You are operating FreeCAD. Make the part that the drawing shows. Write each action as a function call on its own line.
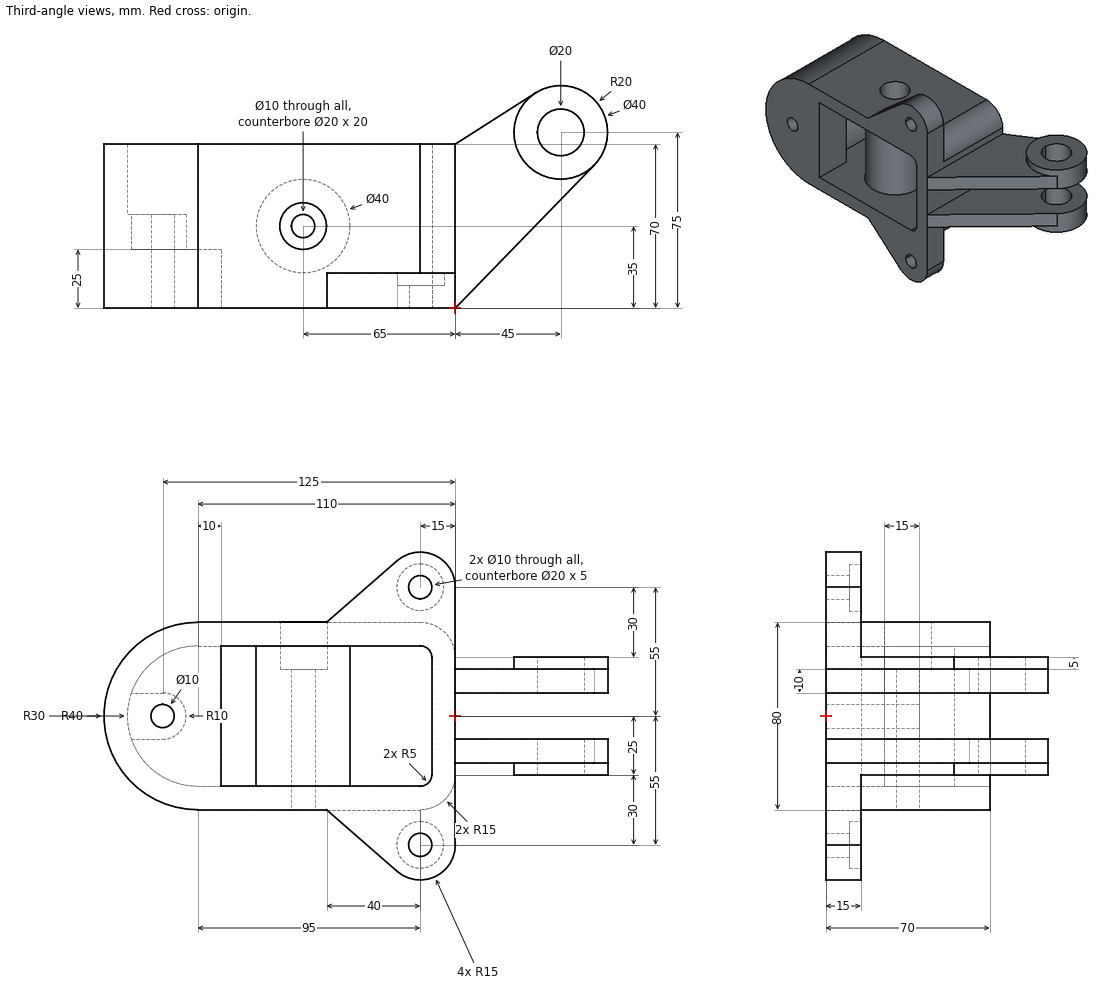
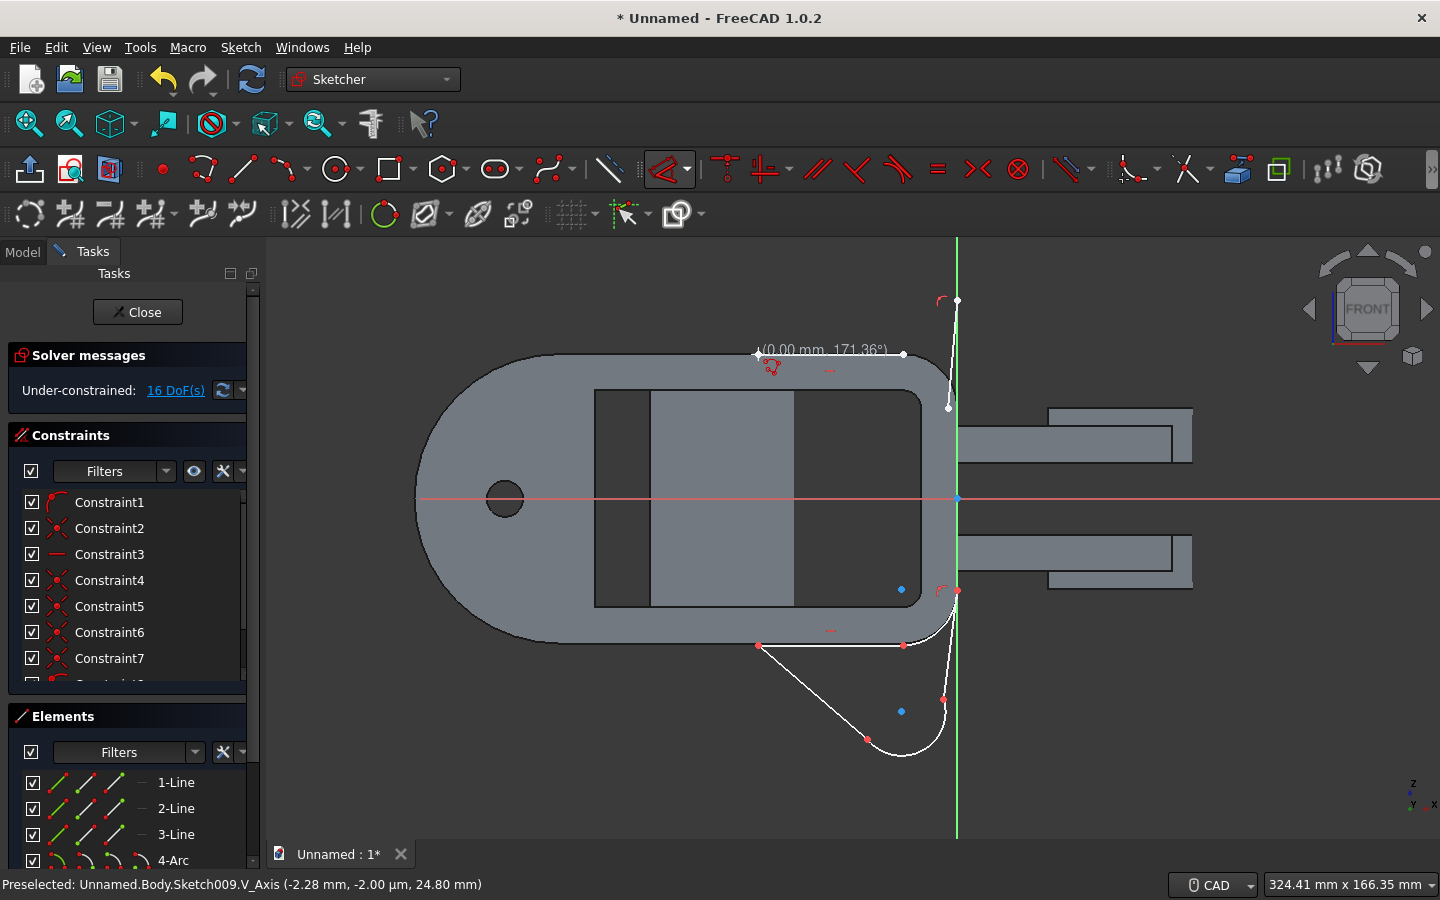
scroll(453, 715, down, 1)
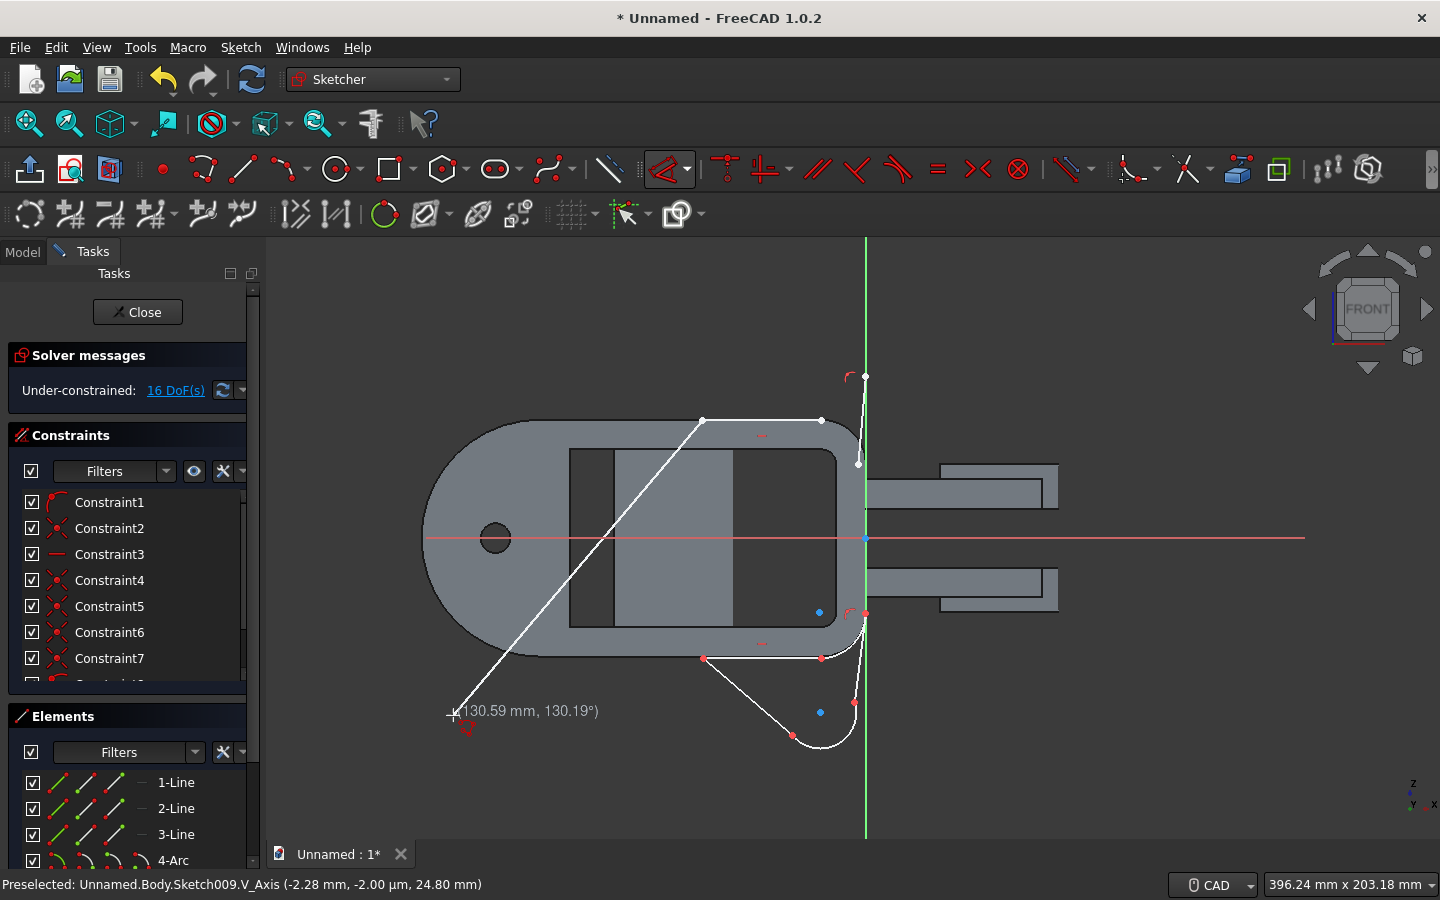
click(792, 342)
right_click(792, 342)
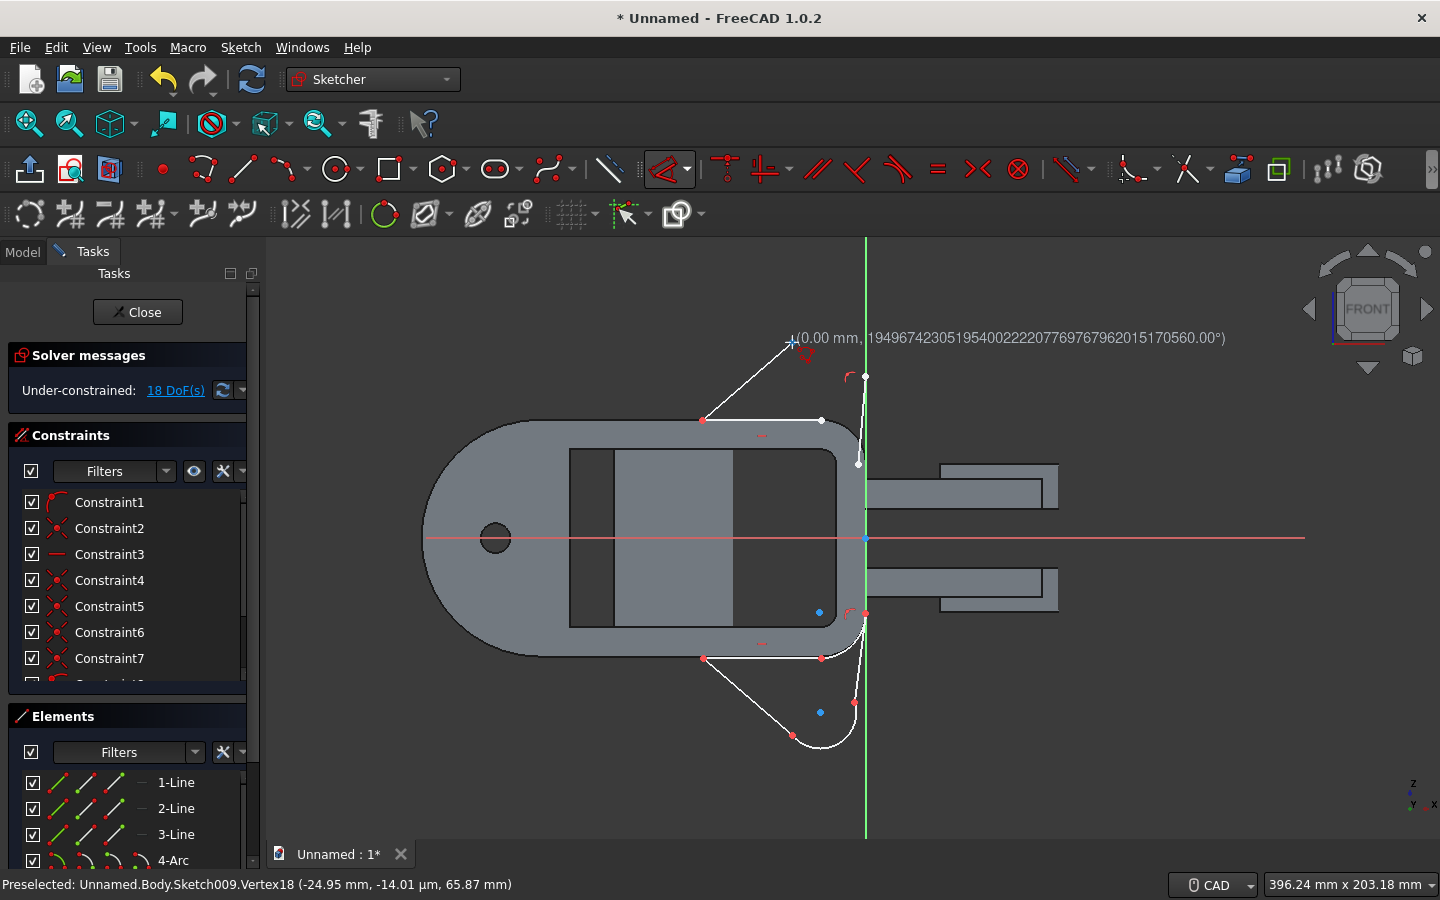
key(g)
key(3)
key(a)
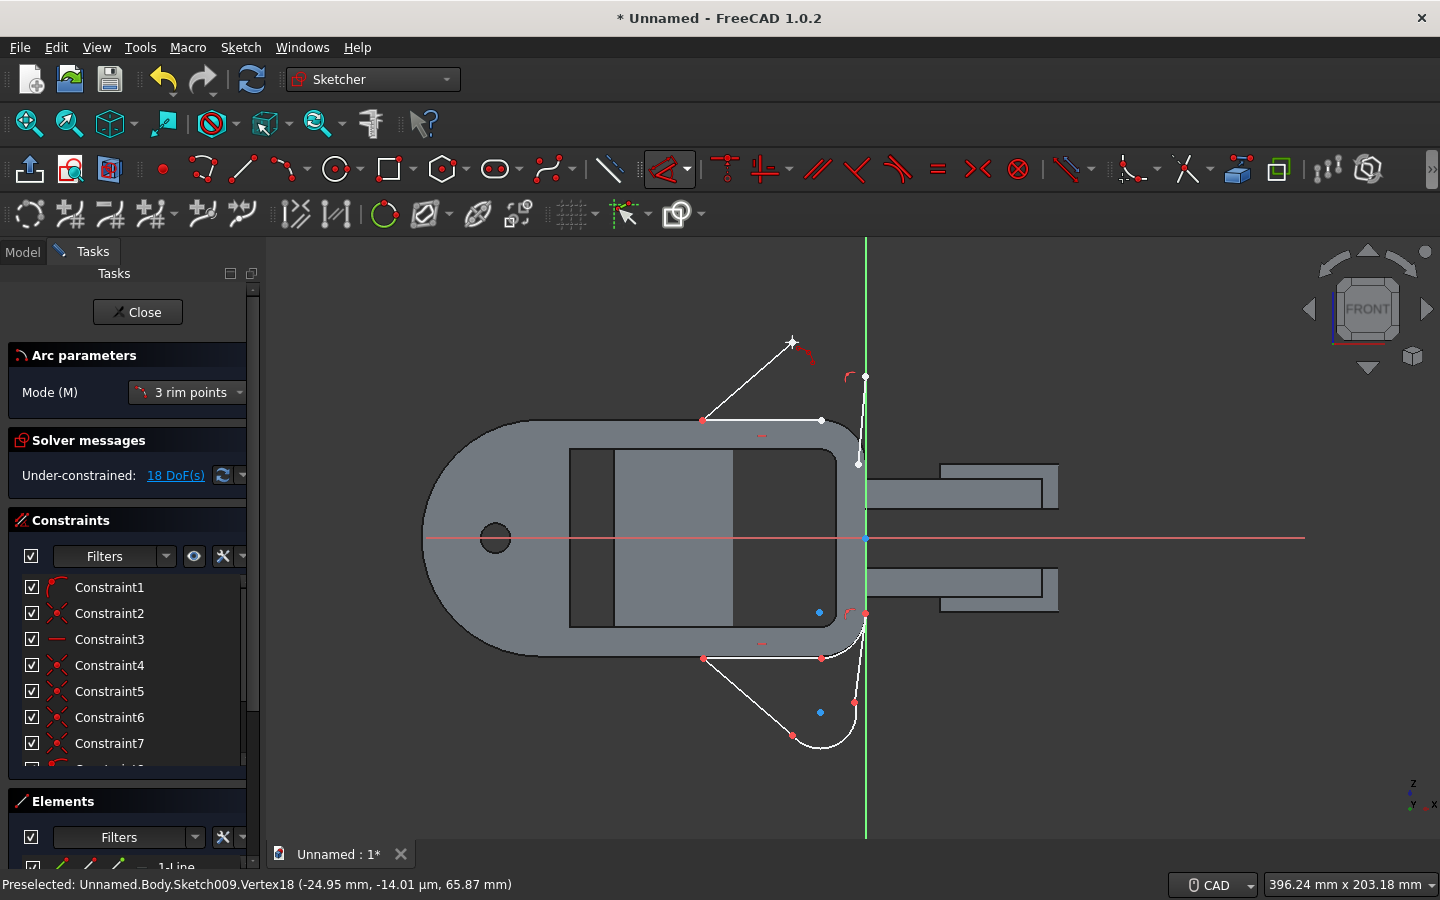
click(858, 465)
click(821, 420)
click(853, 433)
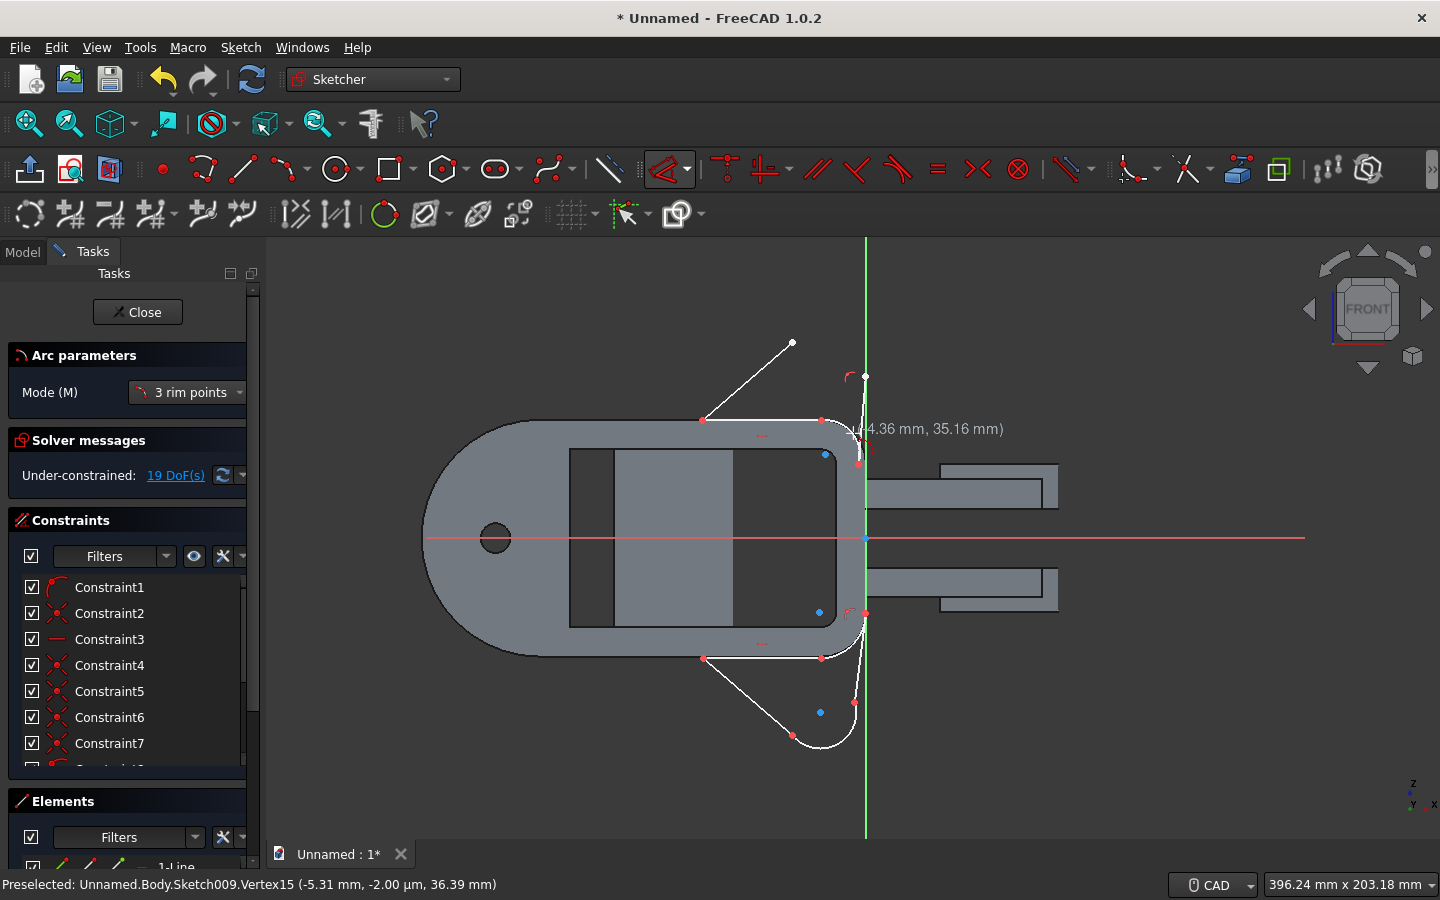
click(792, 343)
click(866, 376)
click(840, 335)
key(Escape)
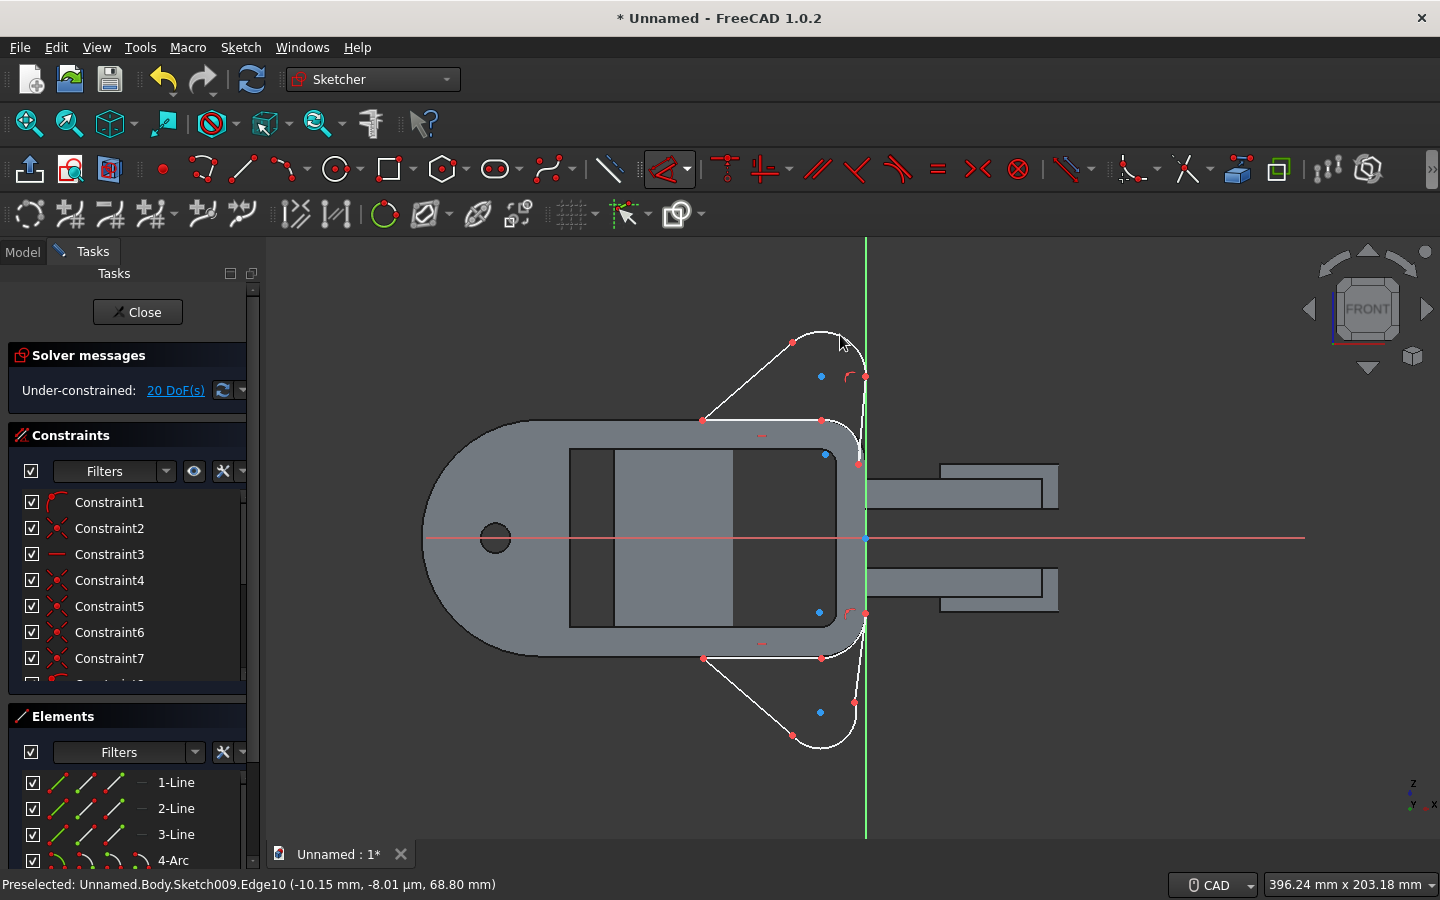
scroll(857, 684, up, 3)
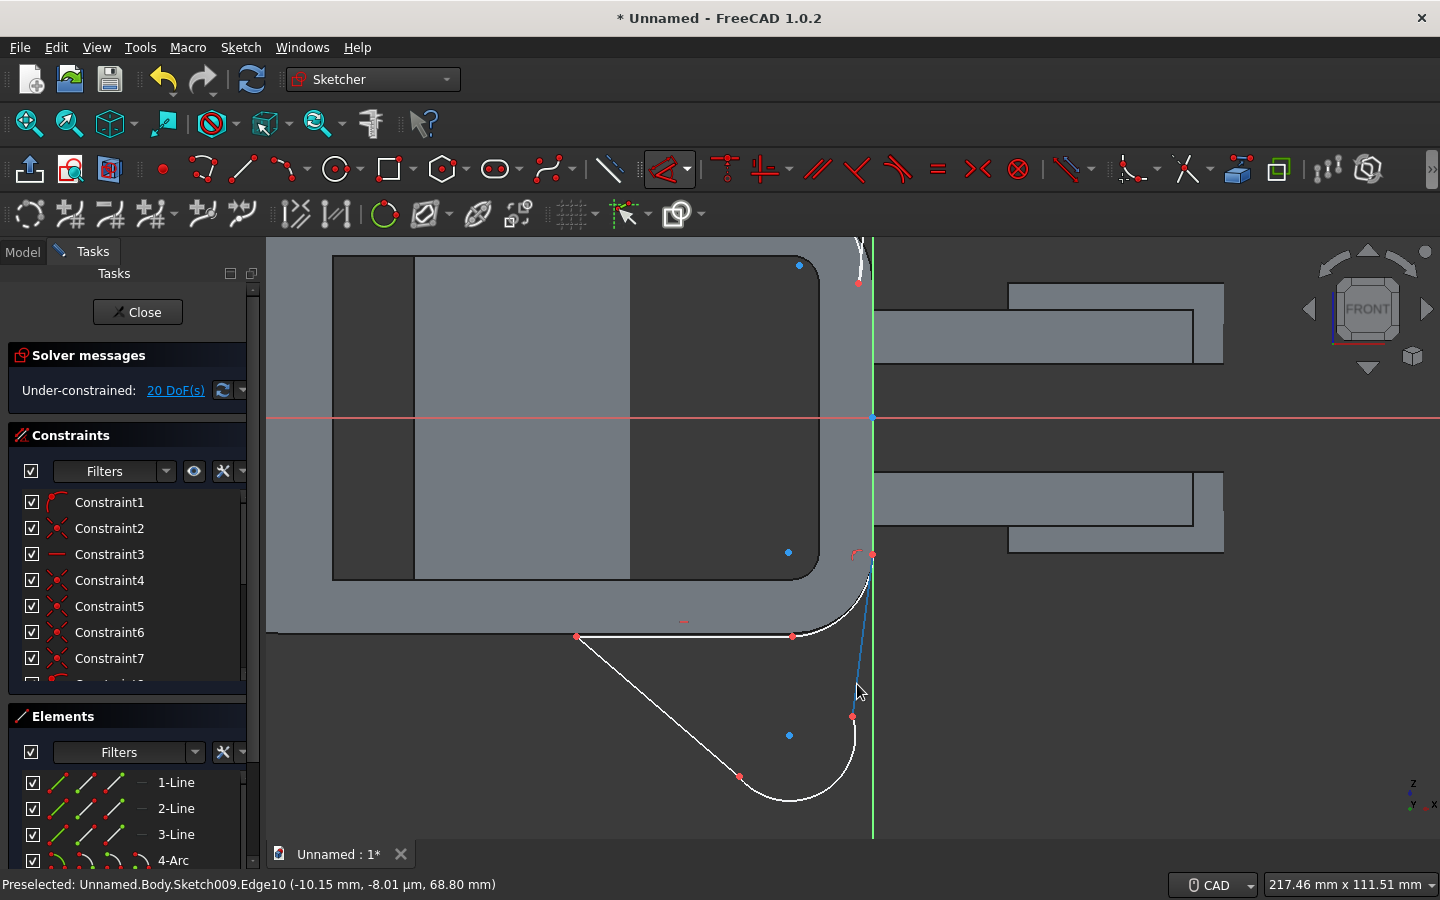
click(857, 684)